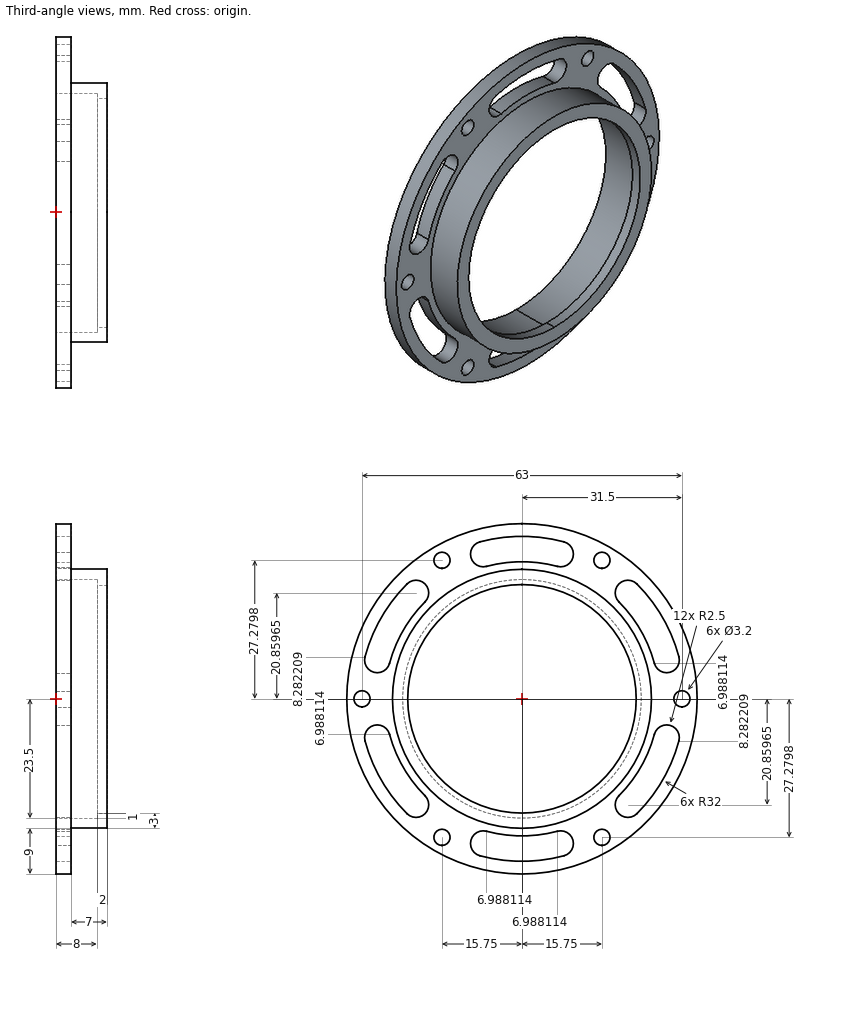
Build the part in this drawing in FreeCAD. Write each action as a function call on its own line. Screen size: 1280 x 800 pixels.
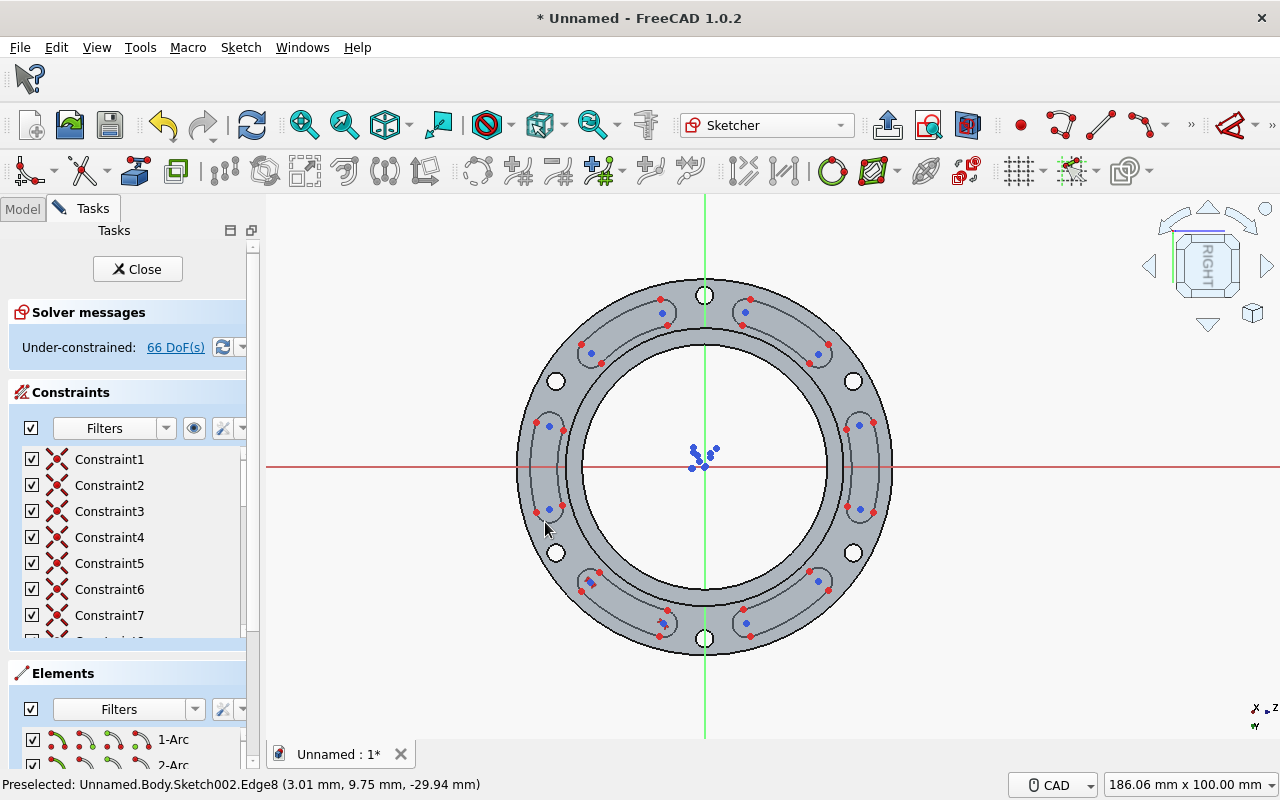
click(561, 418)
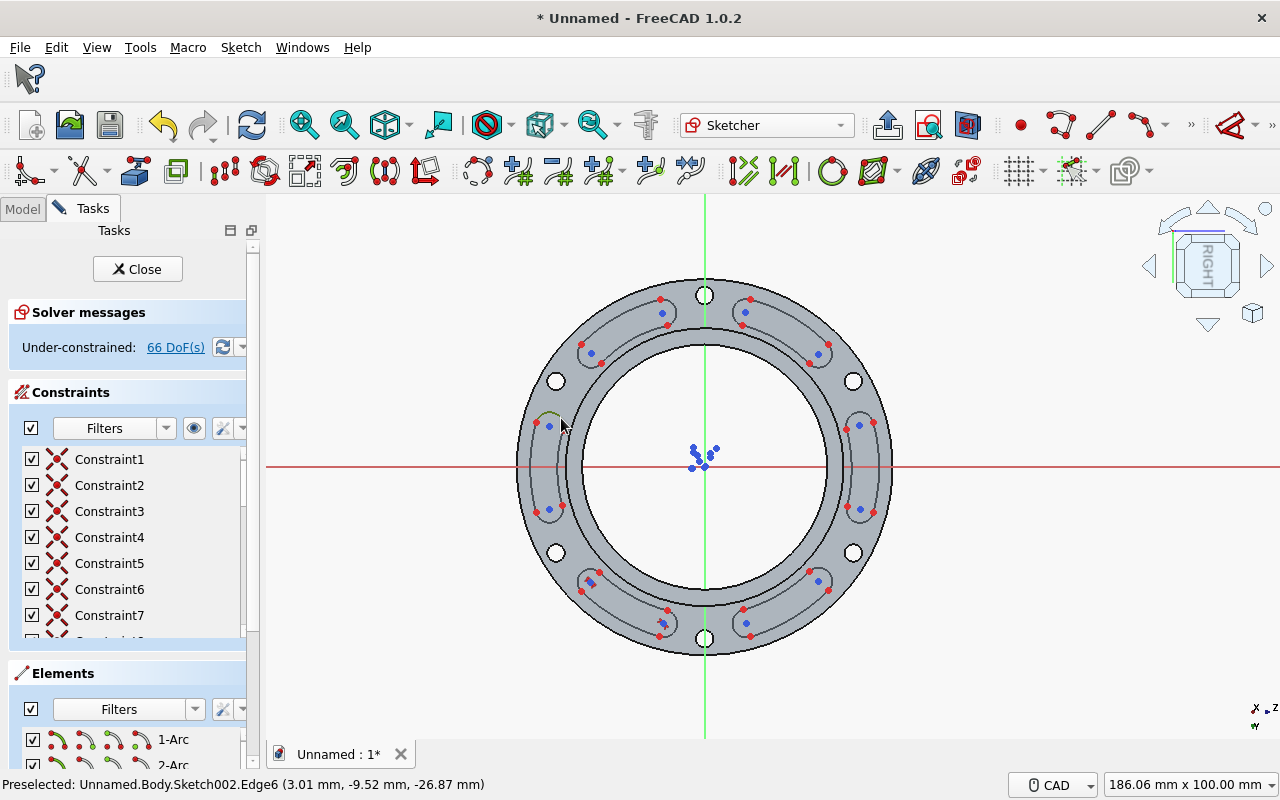
click(531, 449)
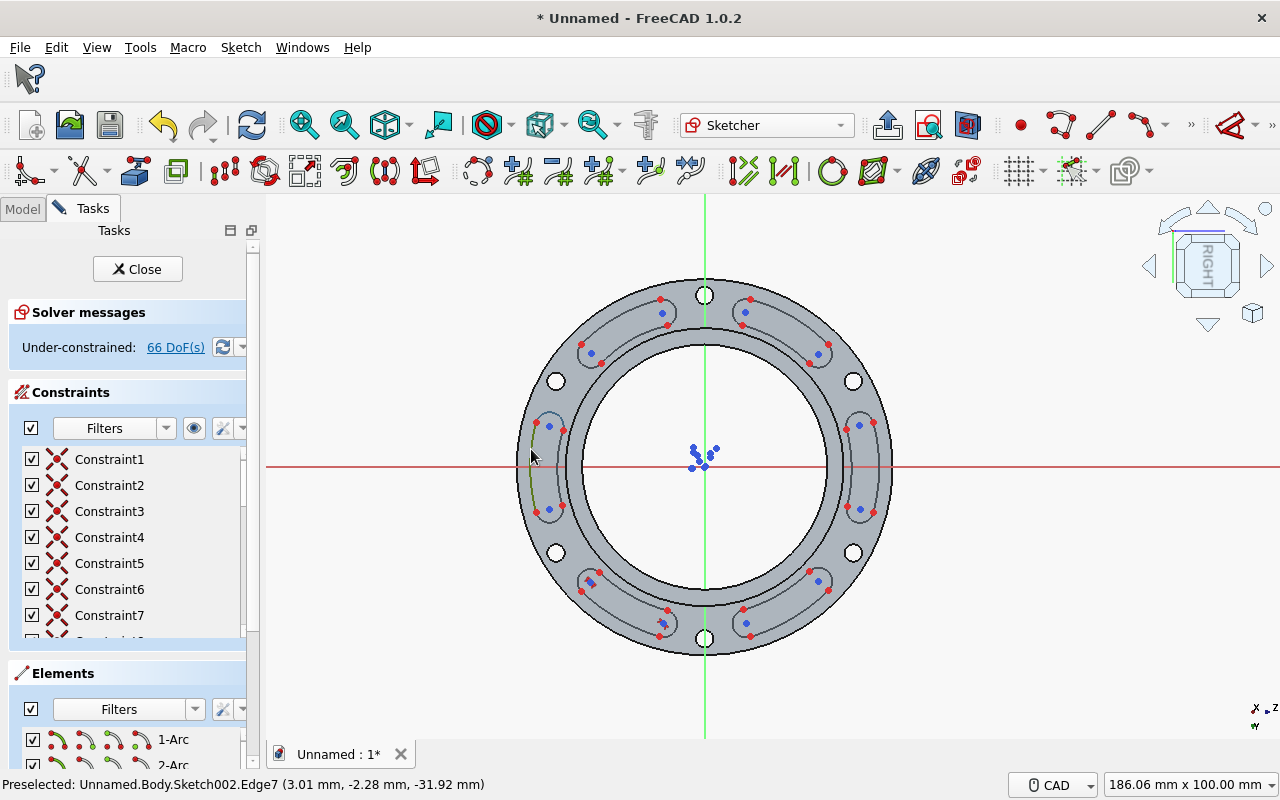
key(t)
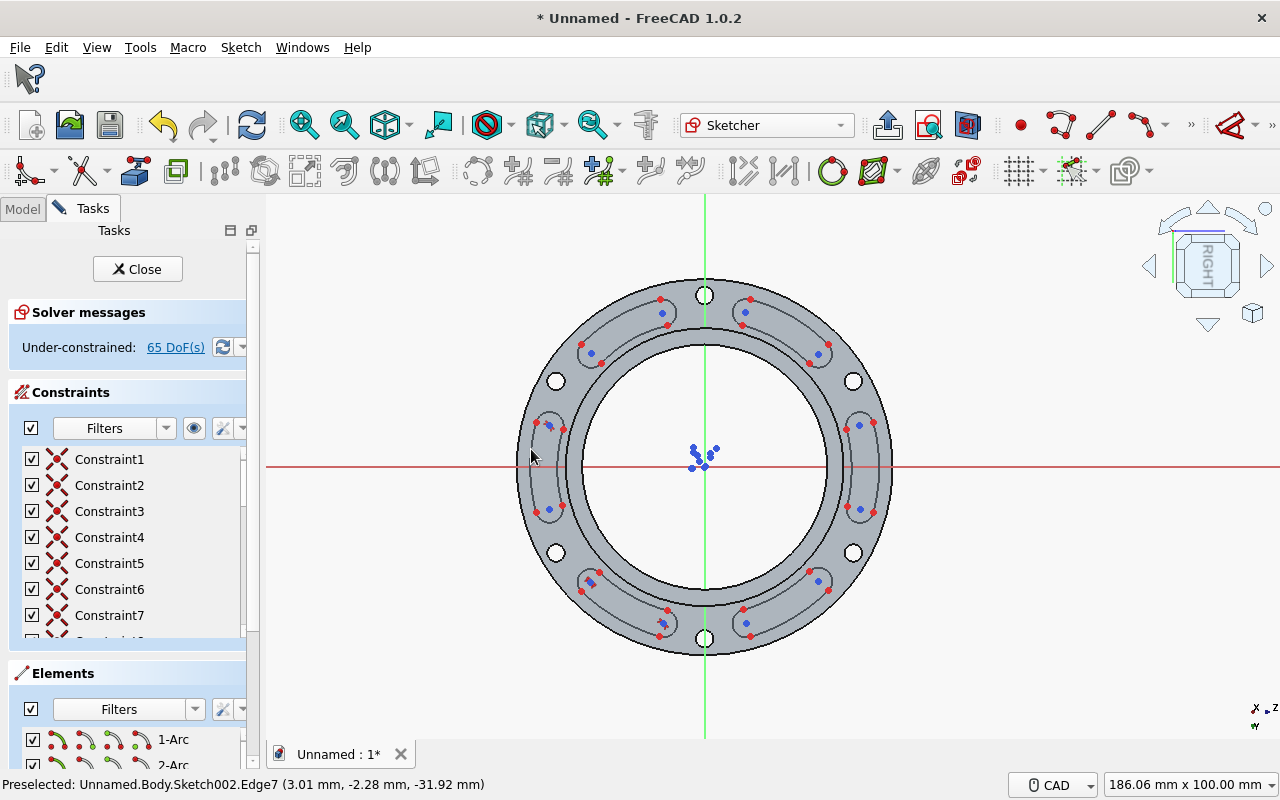
click(531, 449)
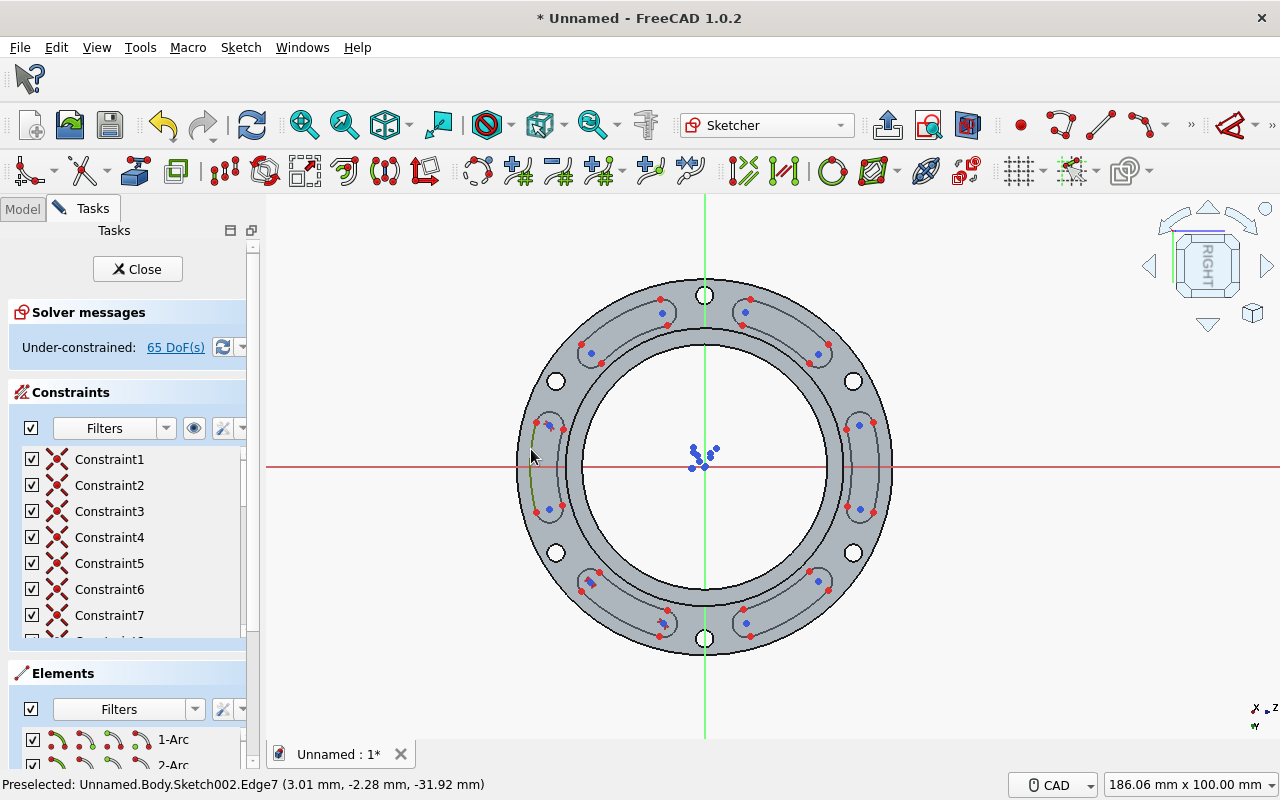
click(544, 522)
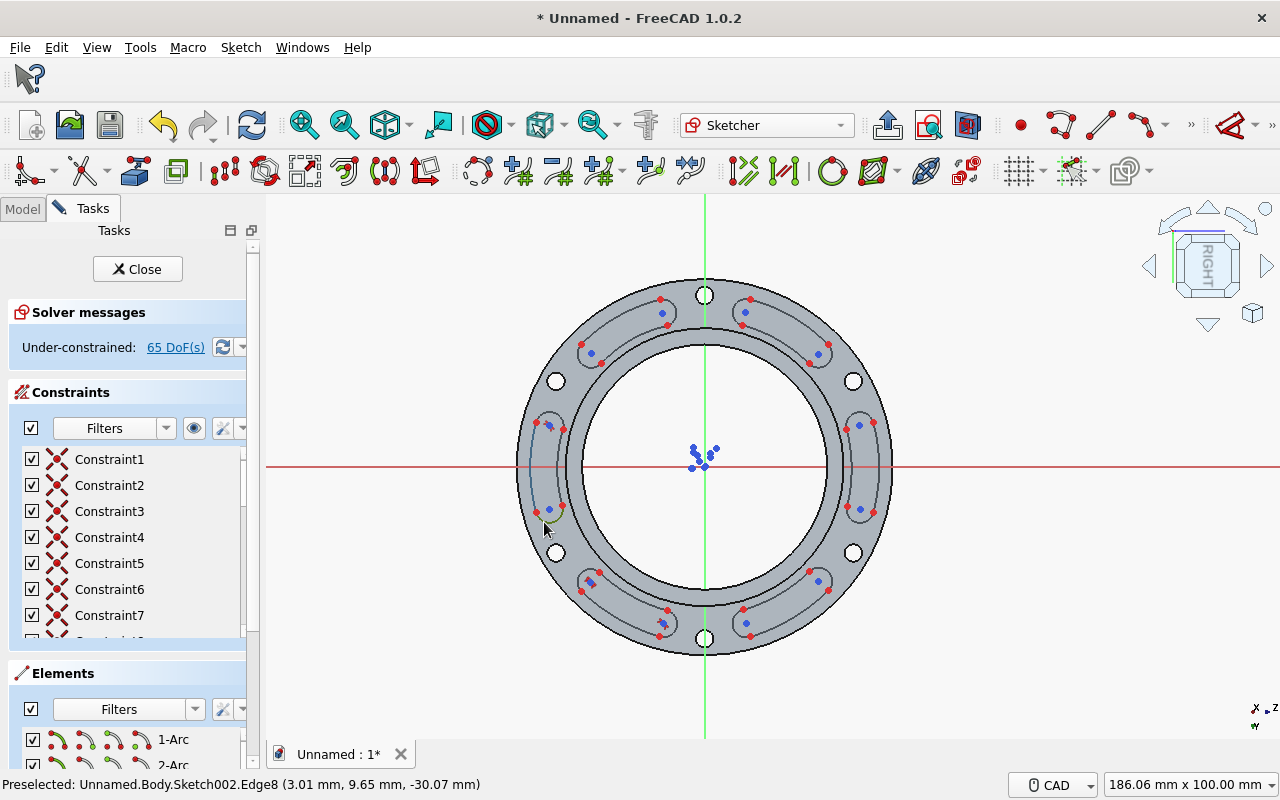
key(t)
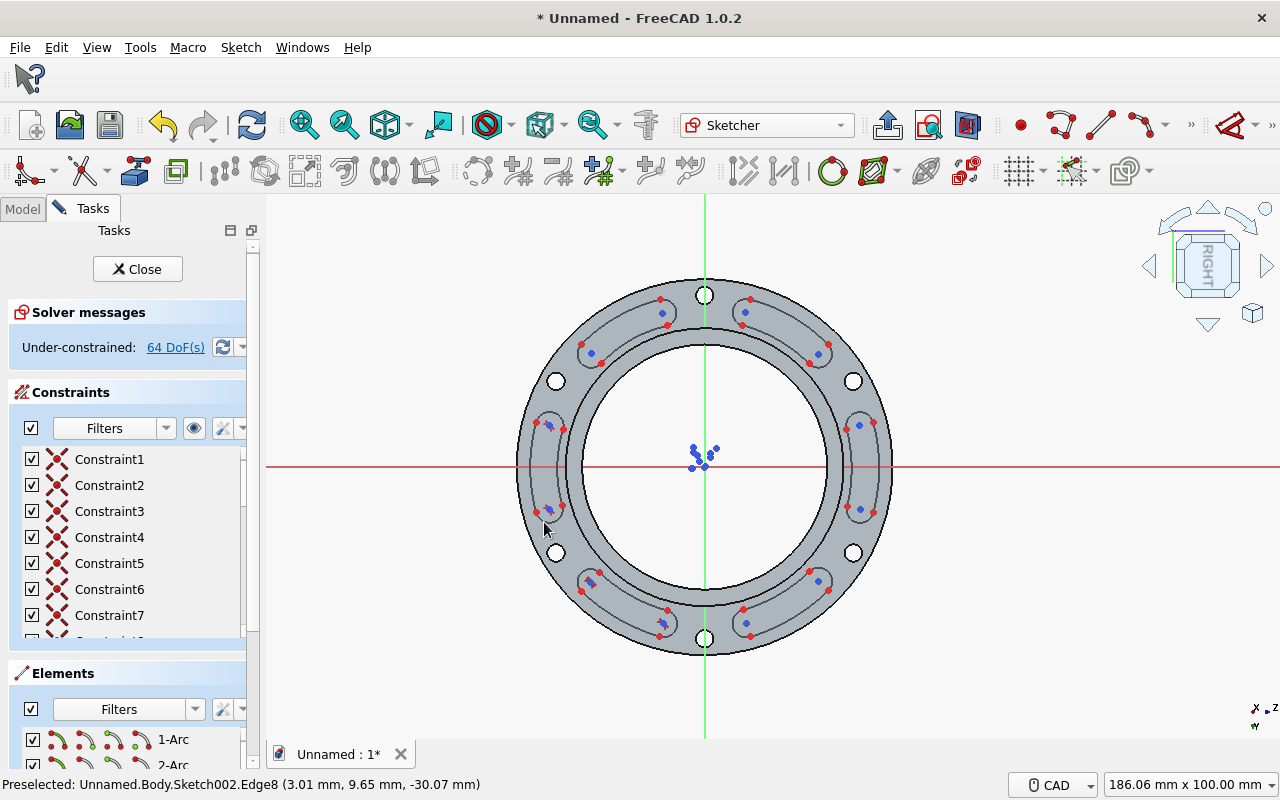
click(645, 333)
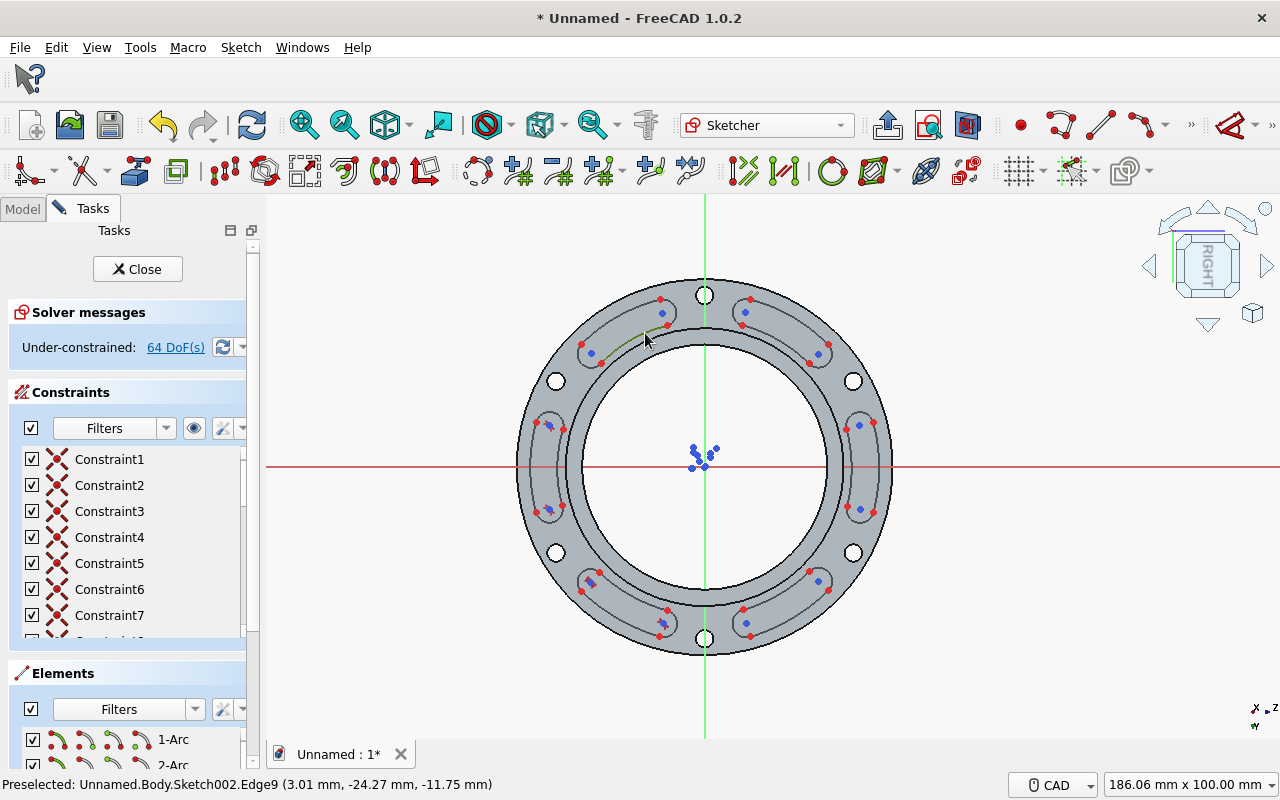
click(676, 318)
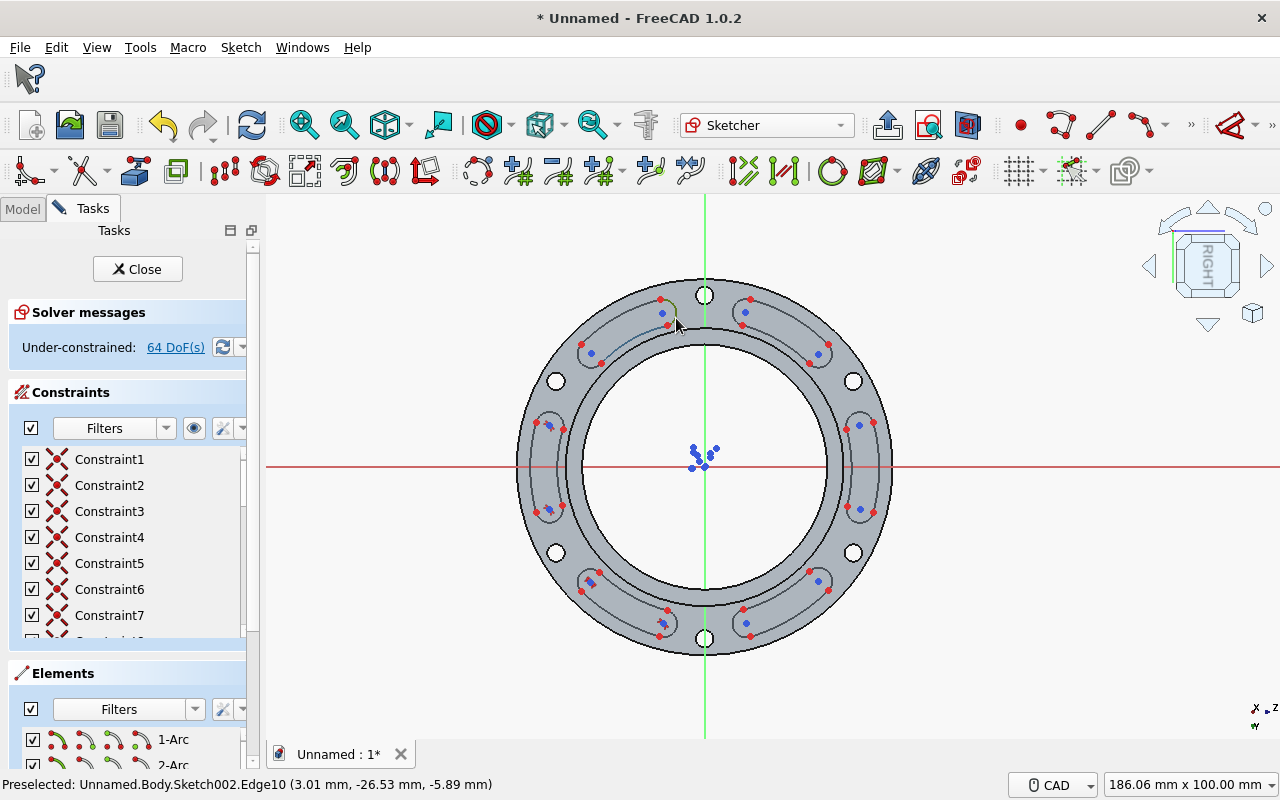
key(t)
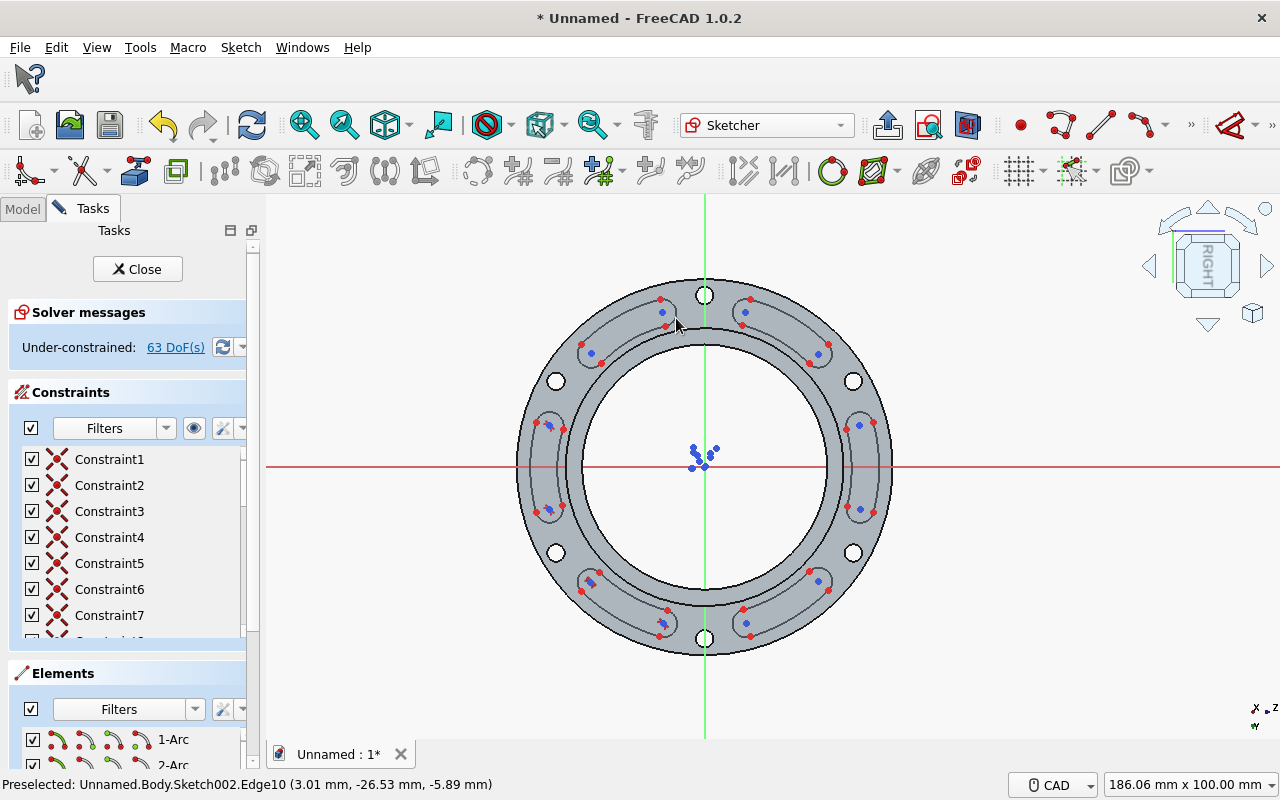
click(644, 333)